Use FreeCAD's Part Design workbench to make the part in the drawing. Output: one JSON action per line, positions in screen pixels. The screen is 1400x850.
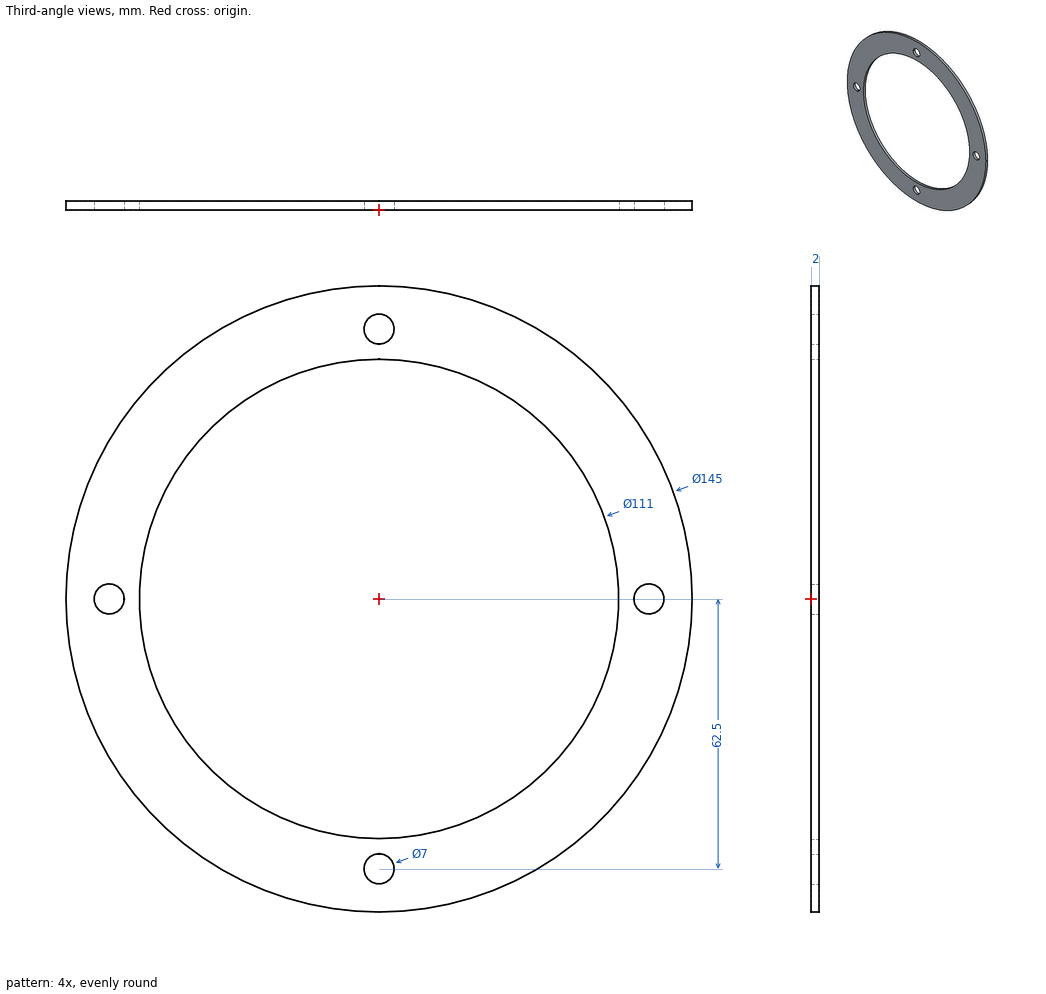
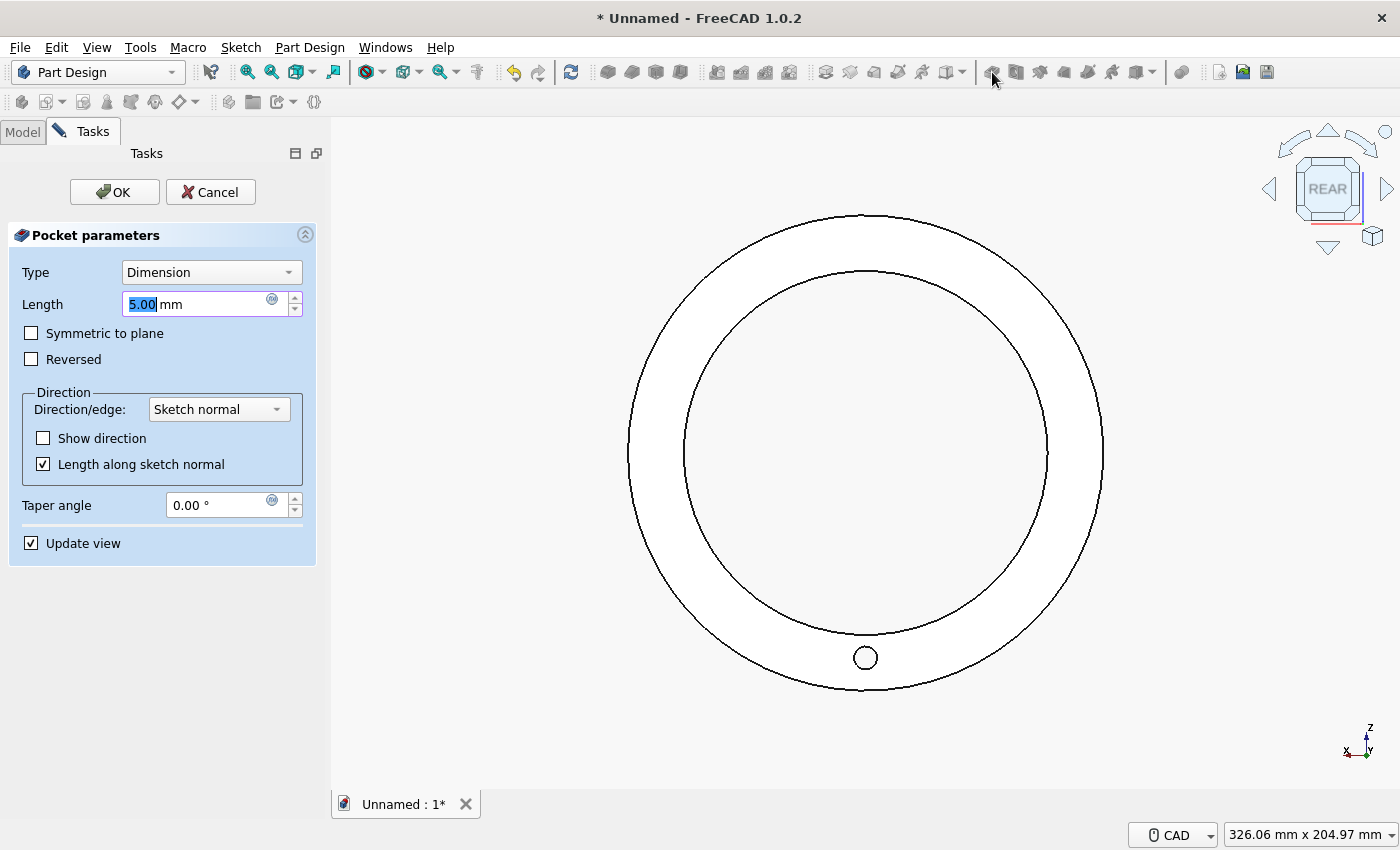
{"action": "left_click", "coordinate": [212, 272]}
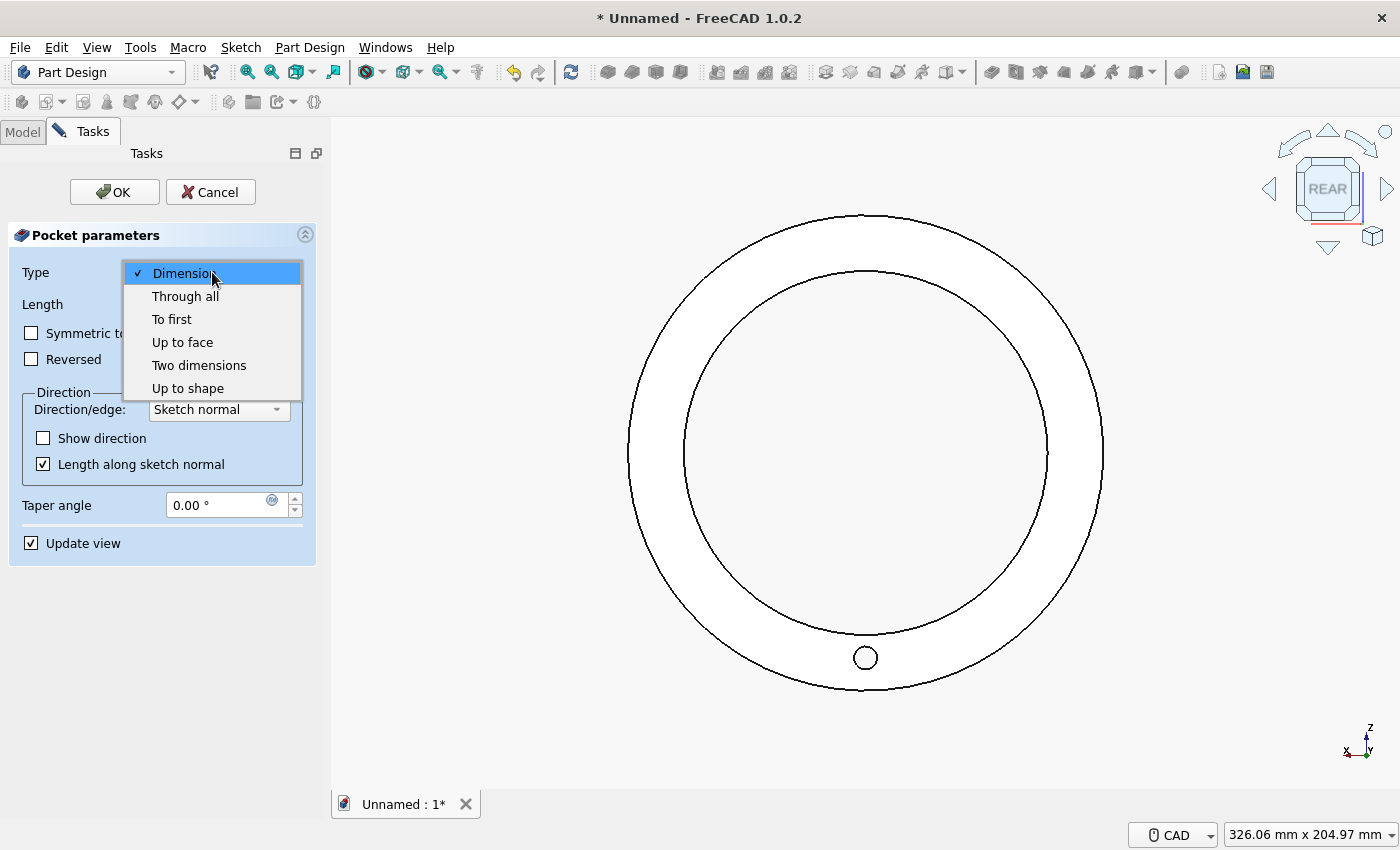
{"action": "left_click", "coordinate": [212, 296]}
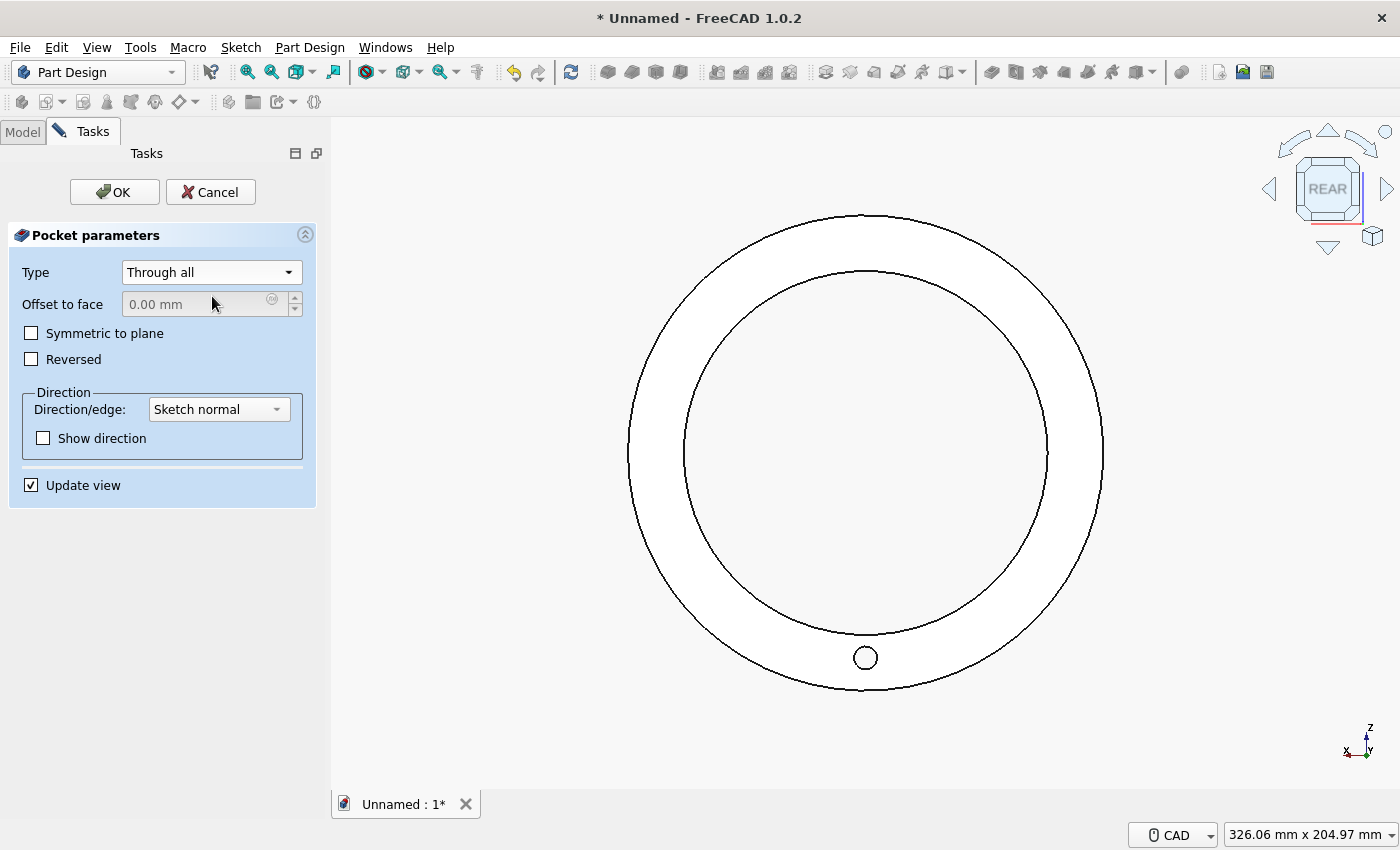
{"action": "left_click", "coordinate": [115, 192]}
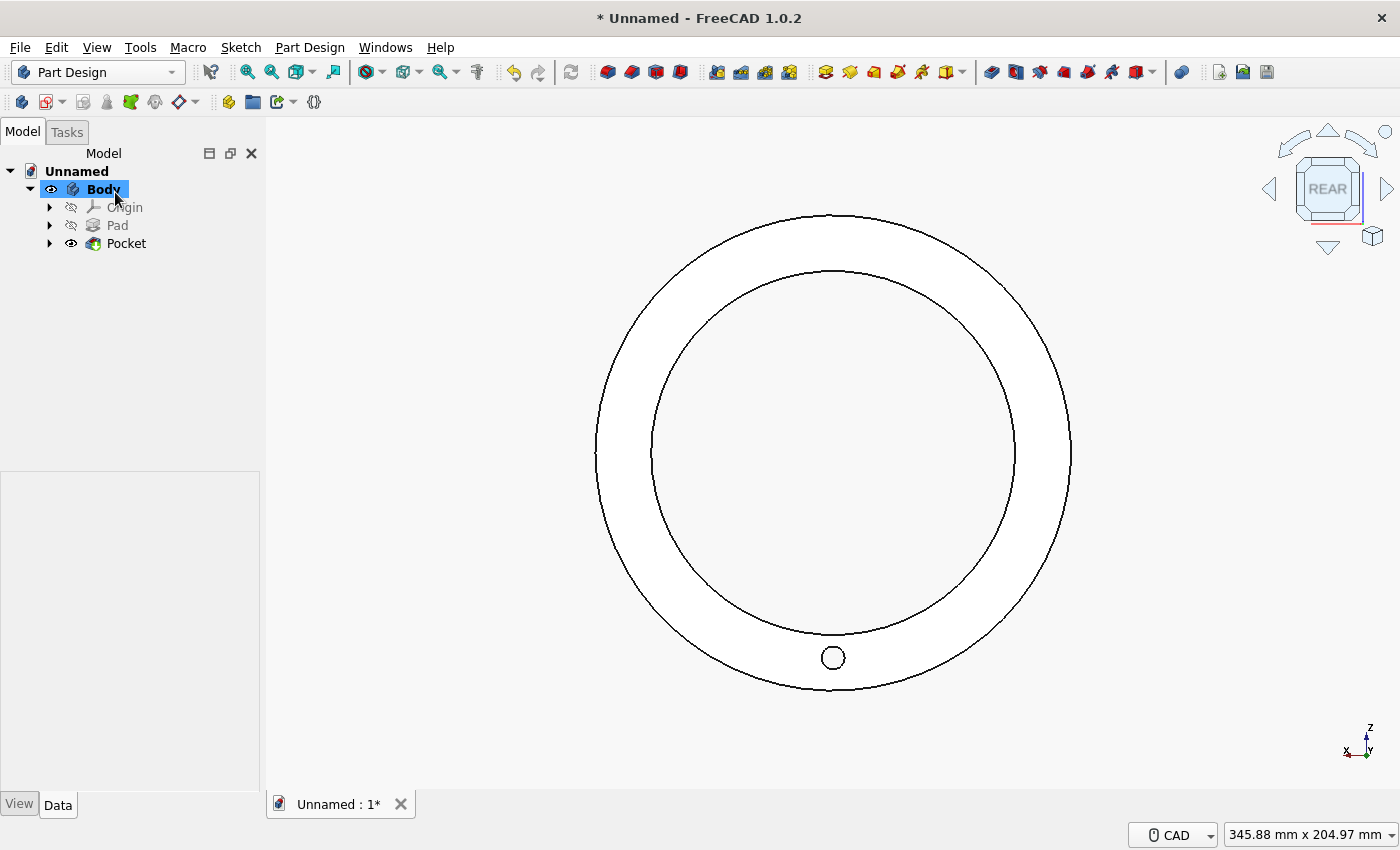
{"action": "left_click", "coordinate": [116, 243]}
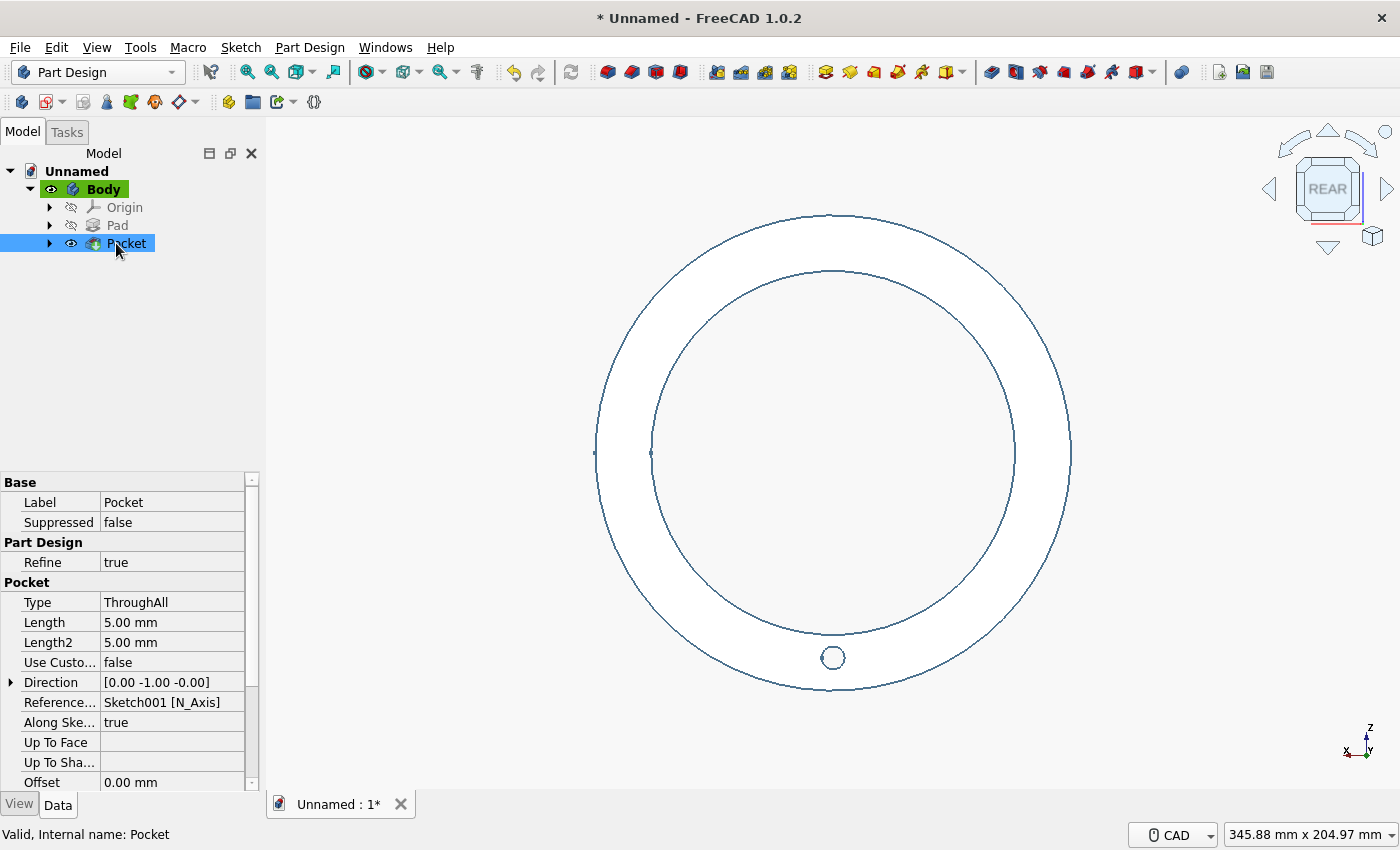
{"action": "left_click", "coordinate": [766, 72]}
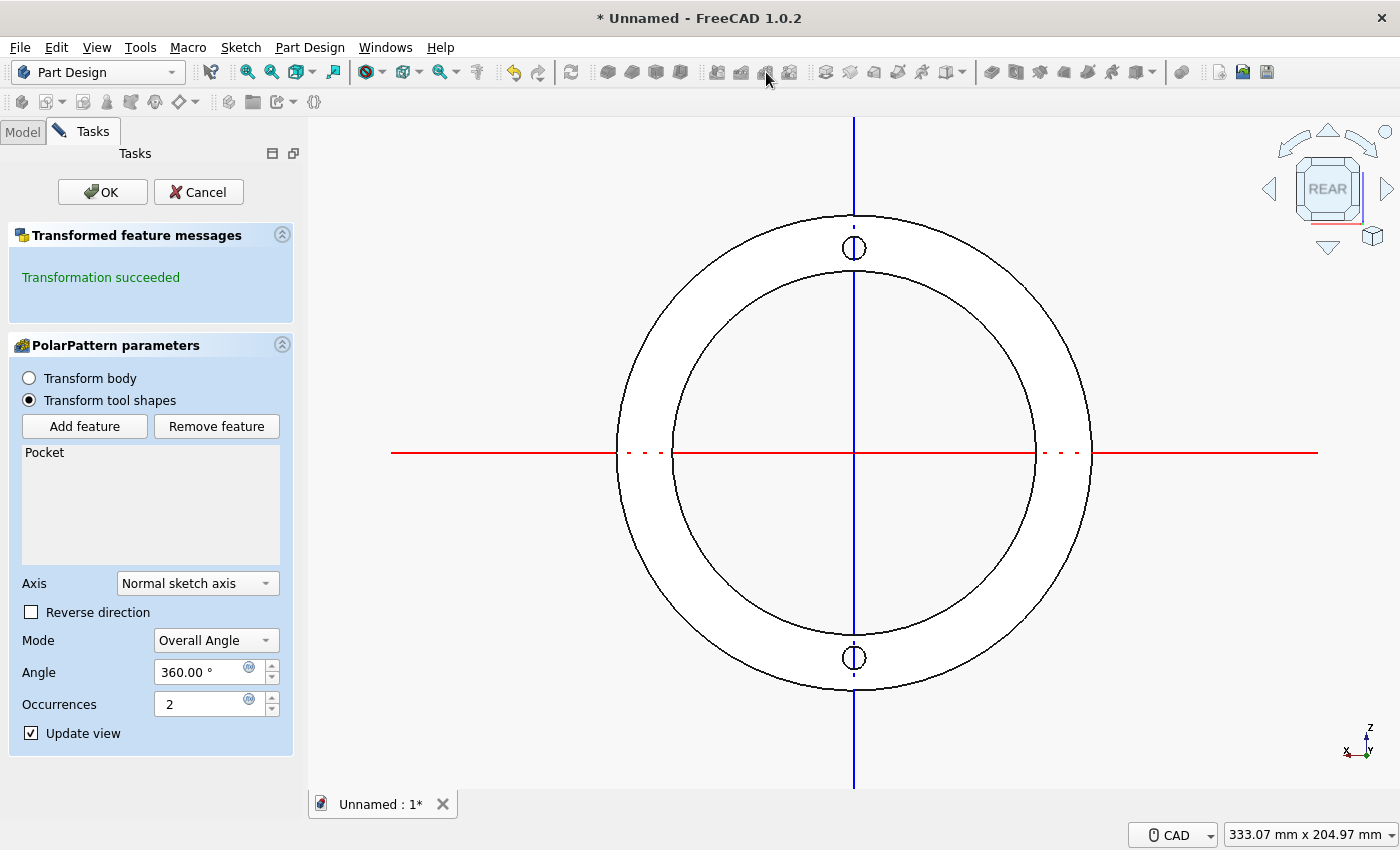
{"action": "left_click", "coordinate": [198, 584]}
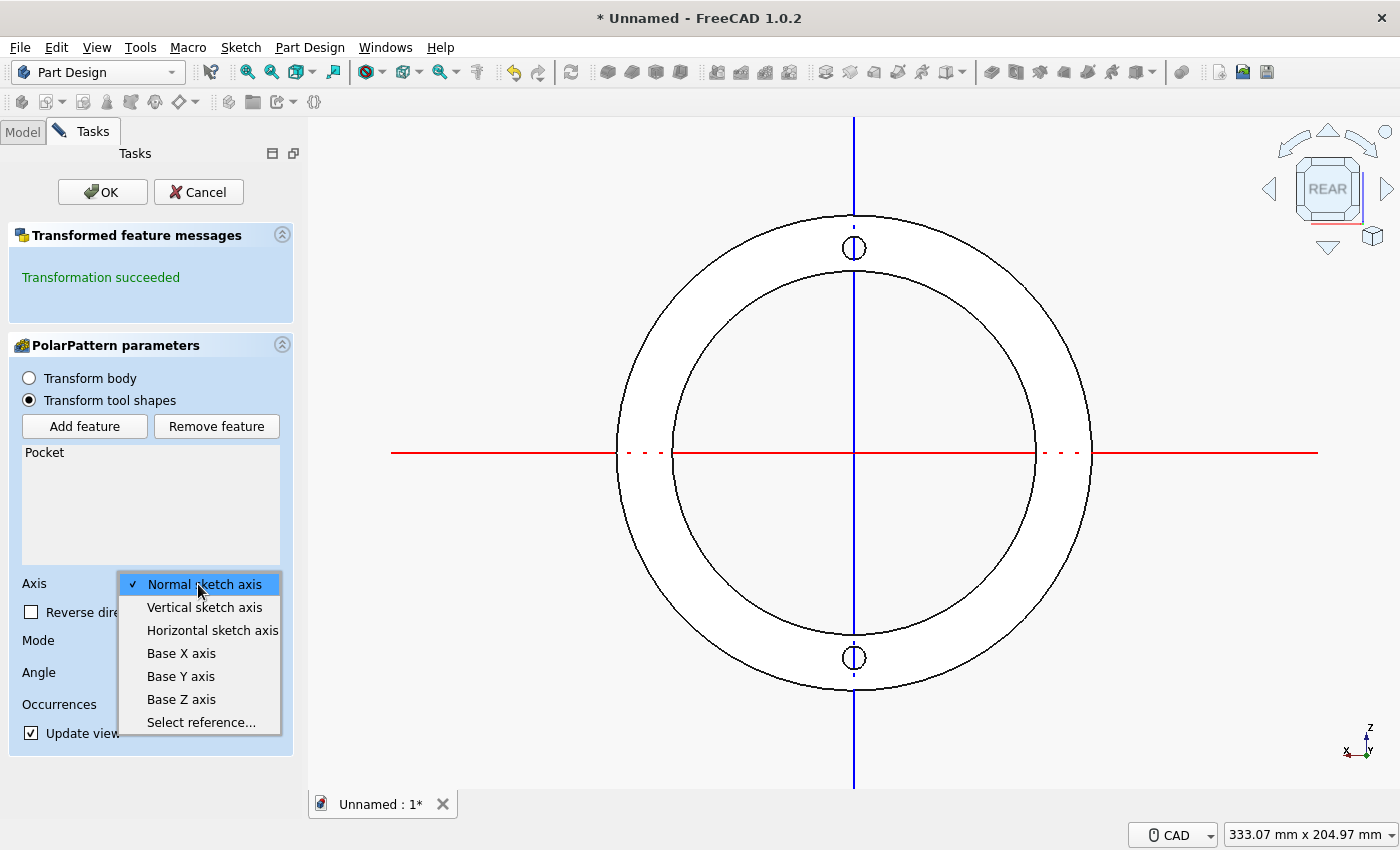
{"action": "left_click", "coordinate": [198, 676]}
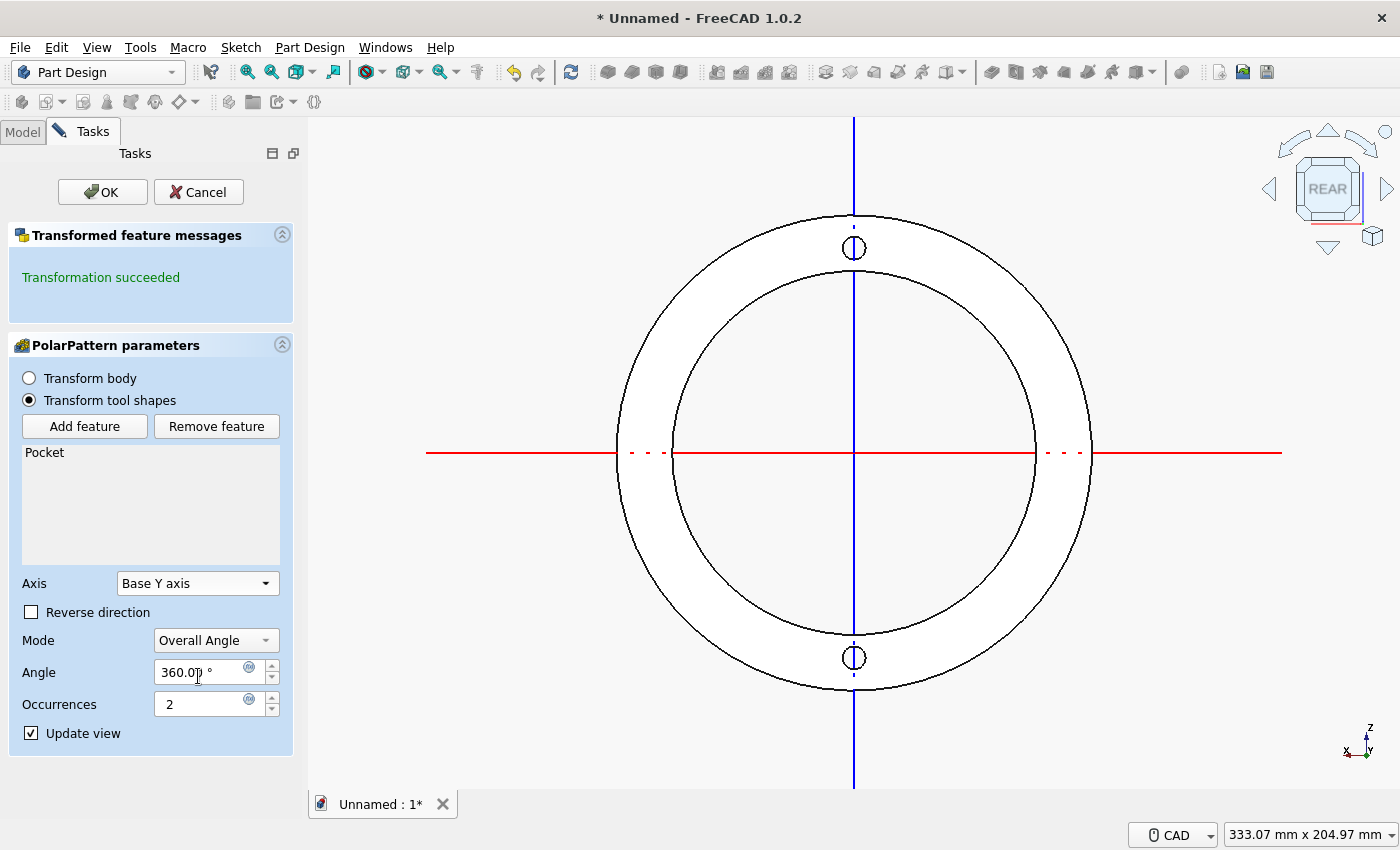
{"action": "triple_click", "coordinate": [209, 704]}